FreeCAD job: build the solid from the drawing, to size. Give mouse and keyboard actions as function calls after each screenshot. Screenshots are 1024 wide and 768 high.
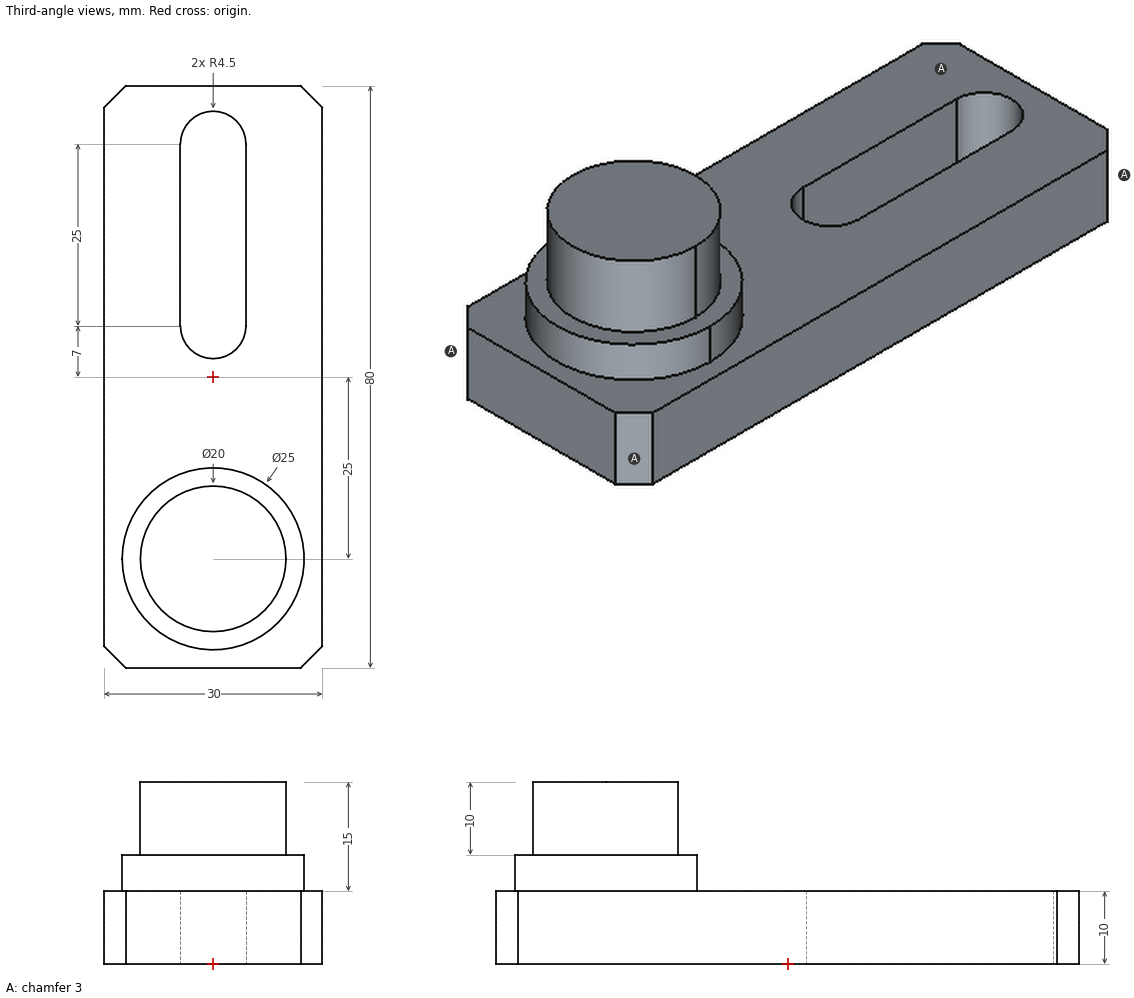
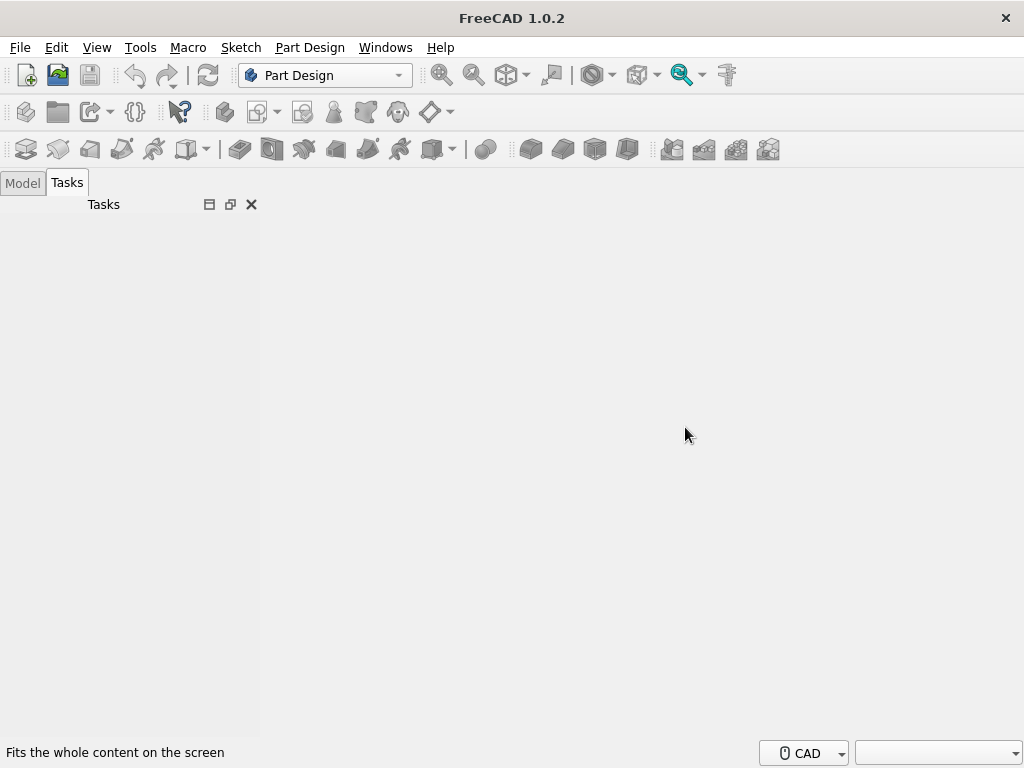
click(26, 76)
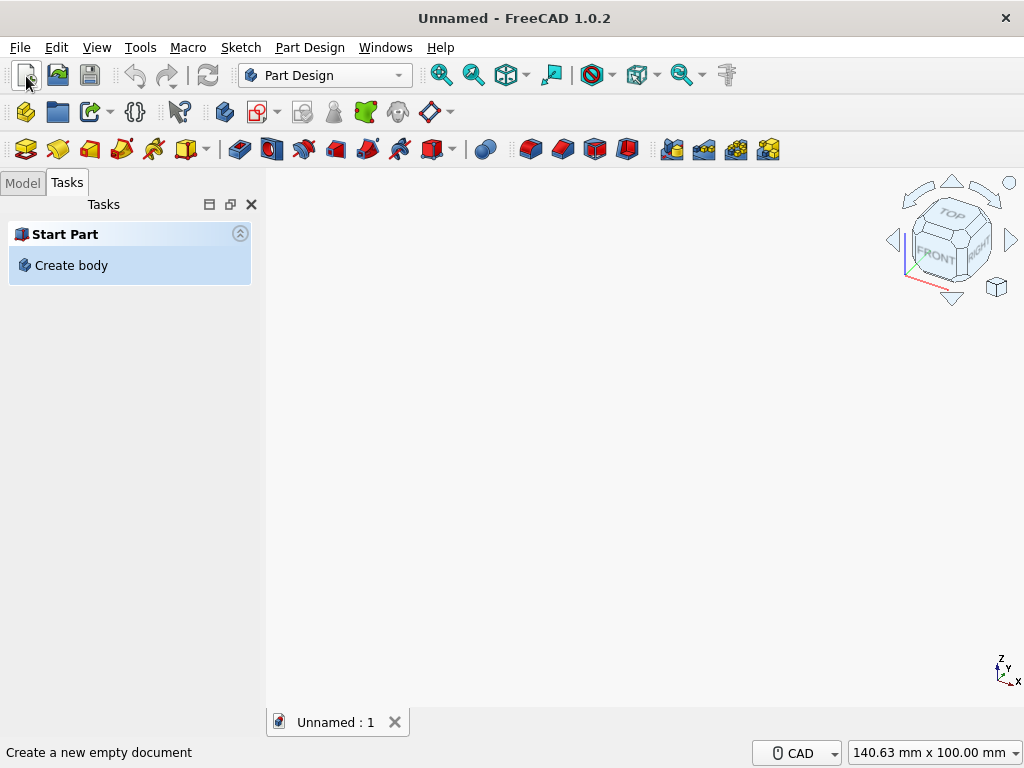
click(258, 112)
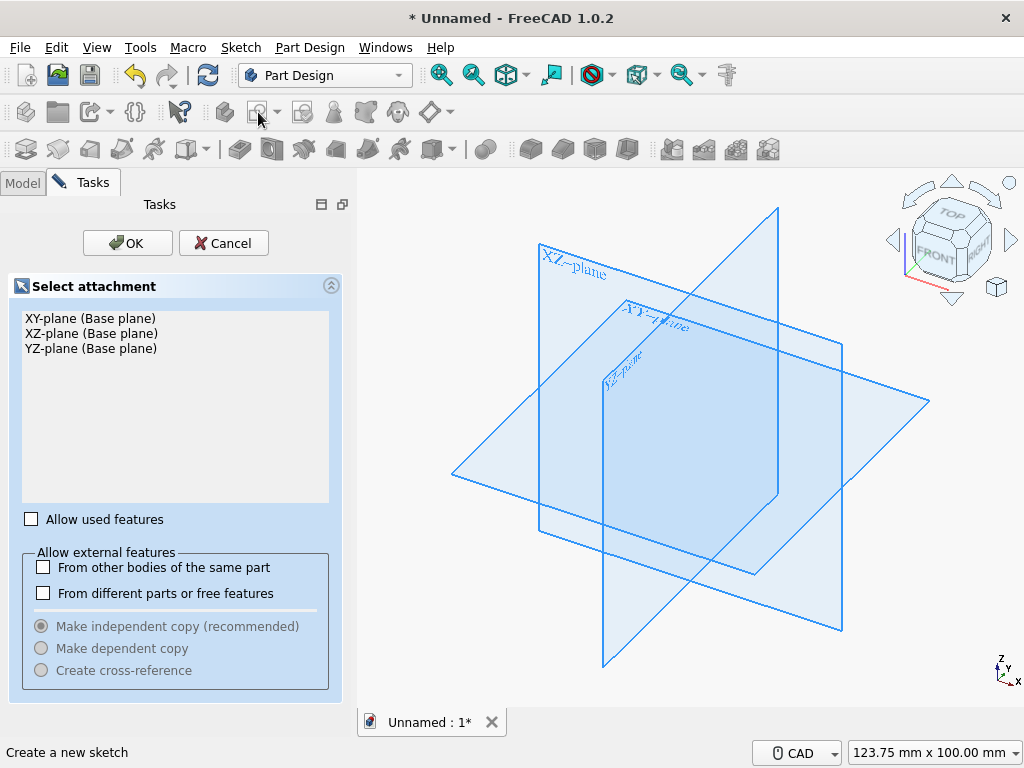
click(82, 318)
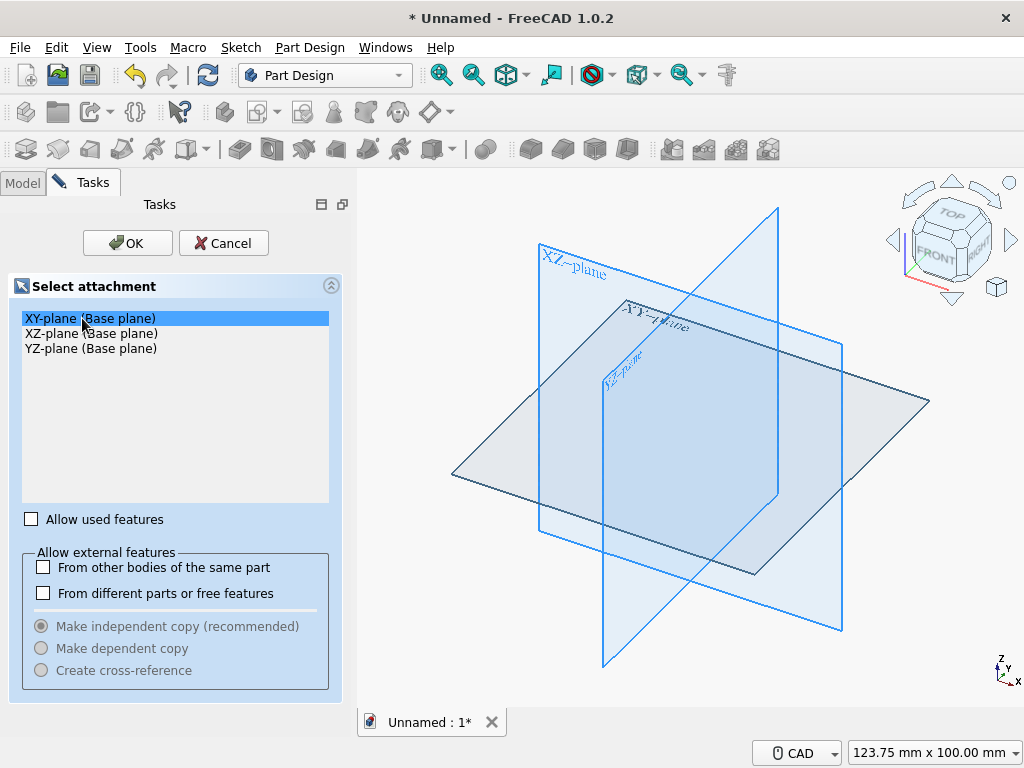
click(128, 243)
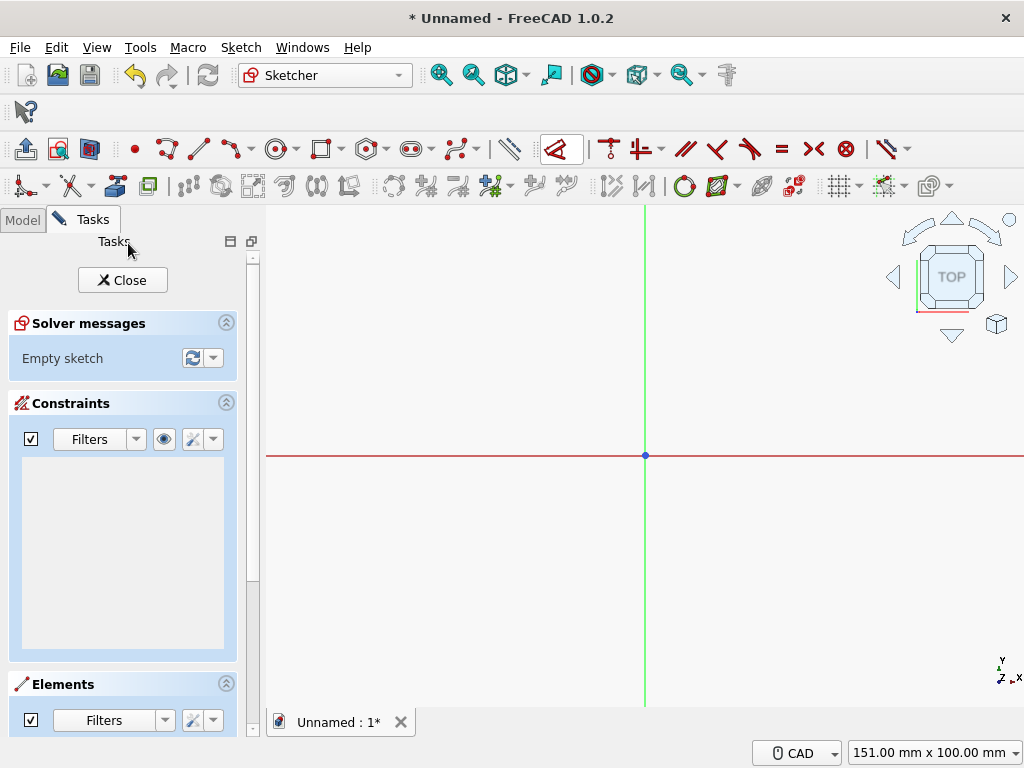
scroll(294, 456, down, 1)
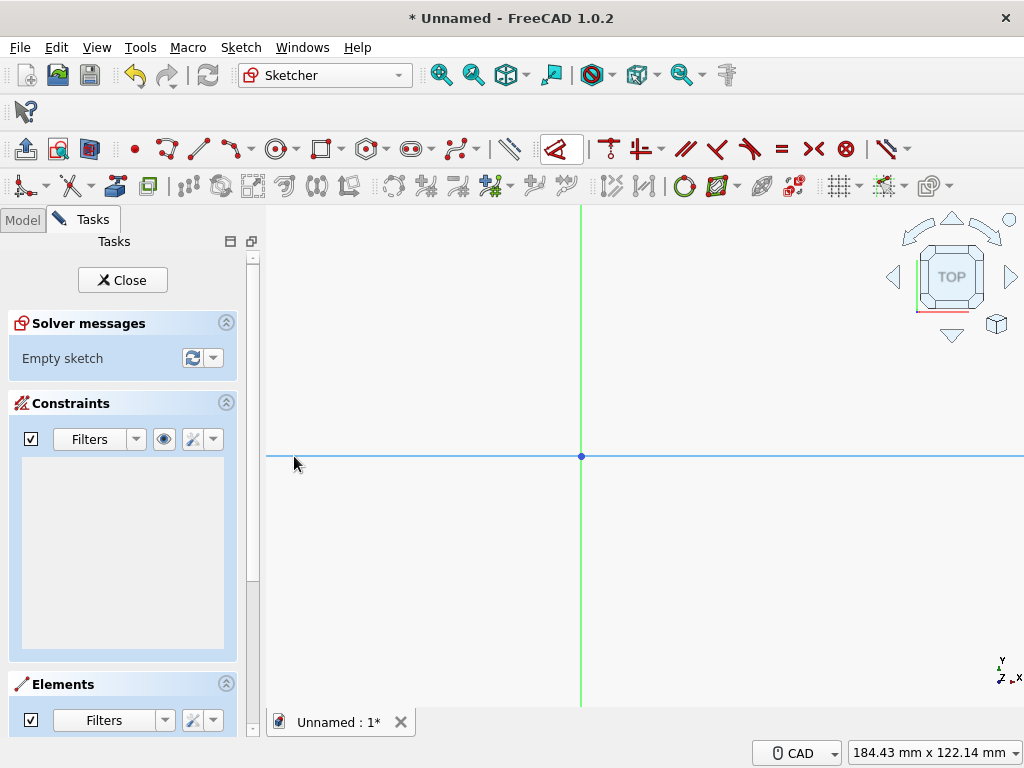
click(344, 150)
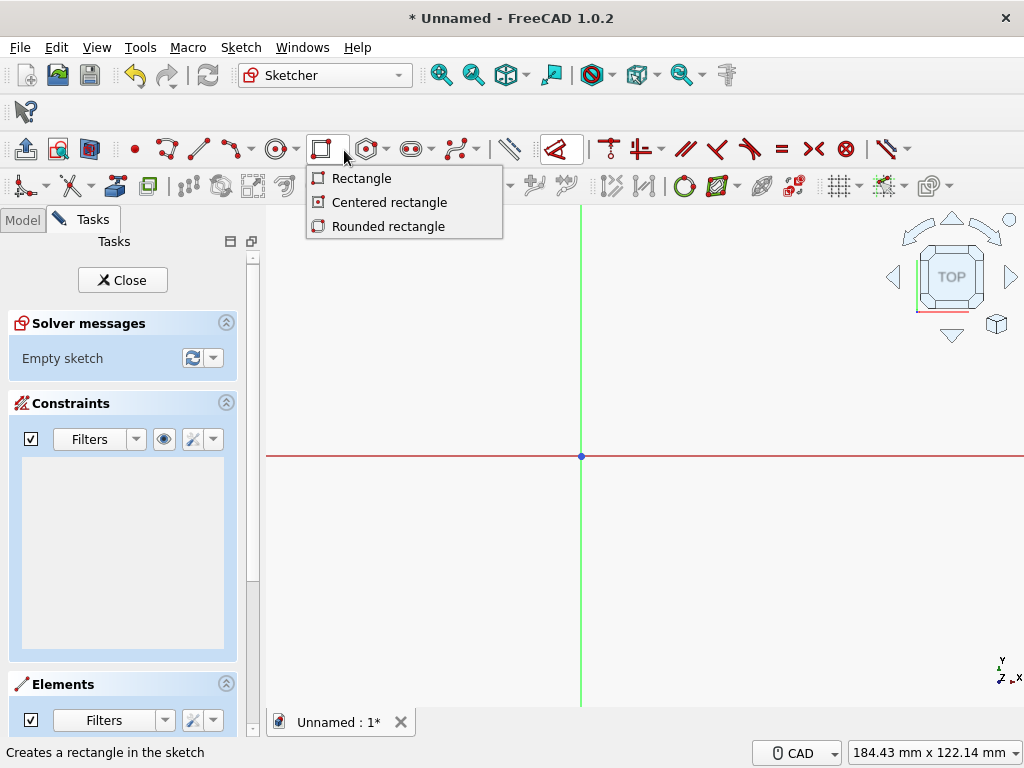
click(404, 202)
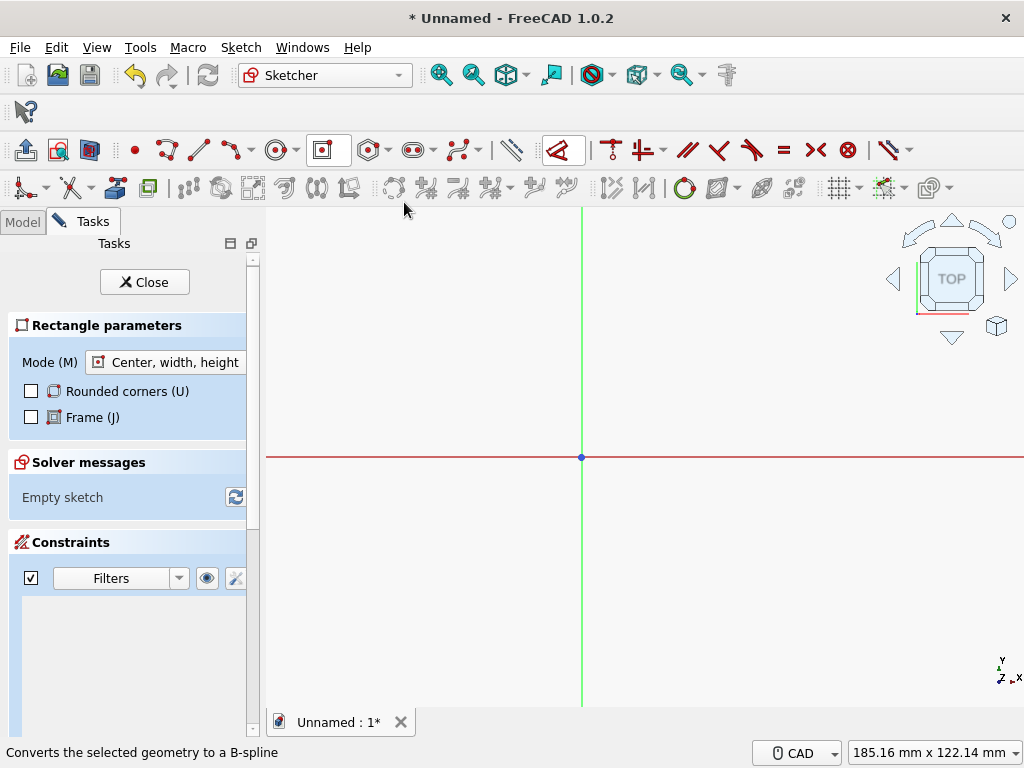
click(582, 457)
move(643, 293)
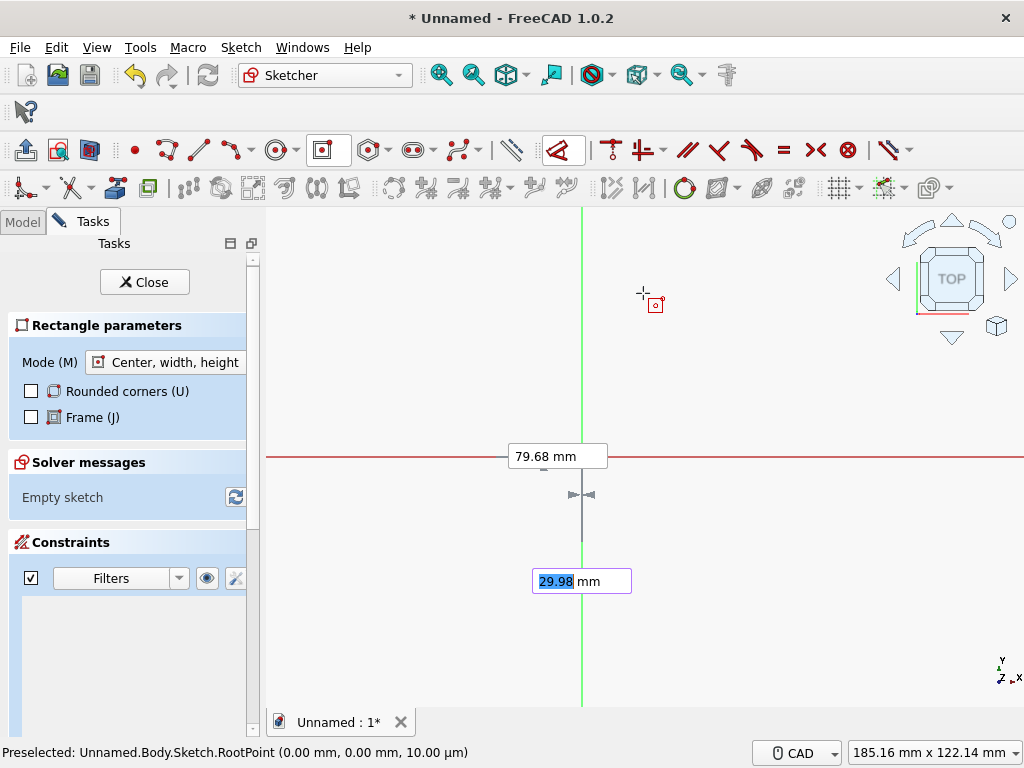
text(30)
key(Tab)
text(80)
key(Return)
key(Escape)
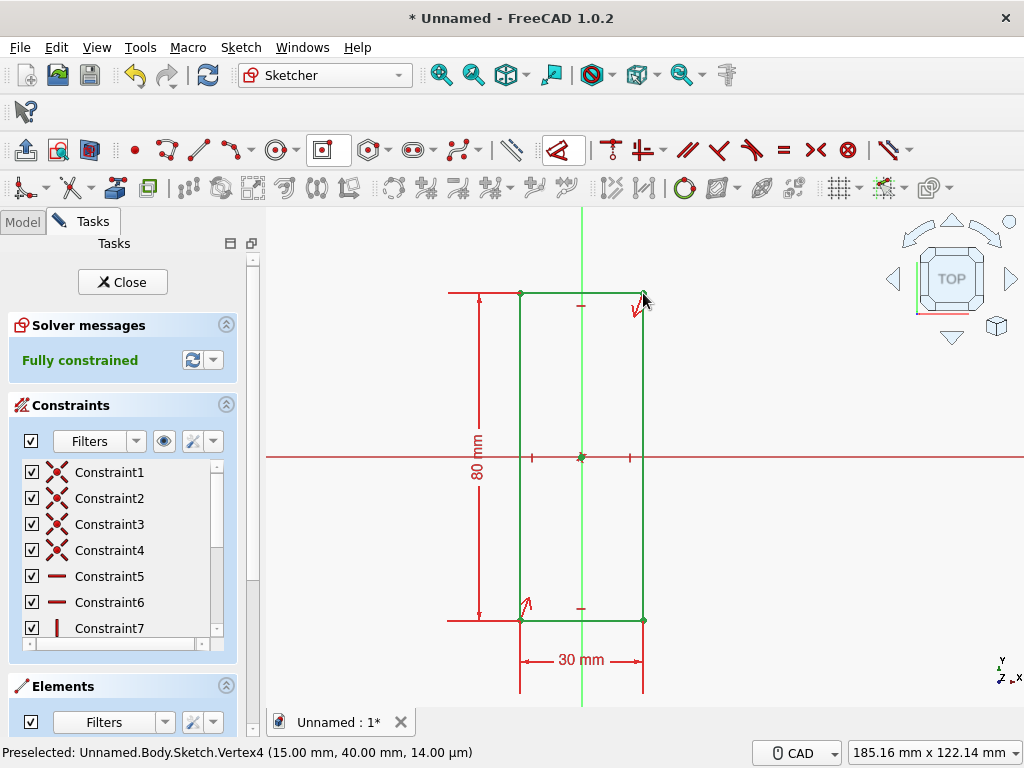
click(123, 282)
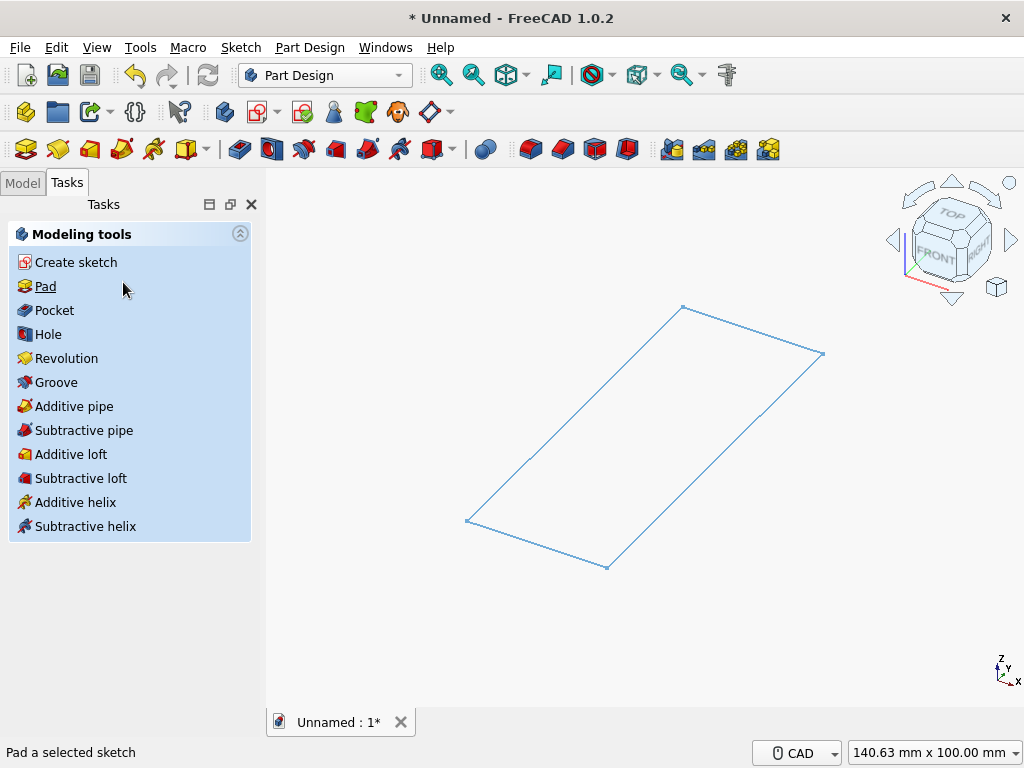
click(26, 150)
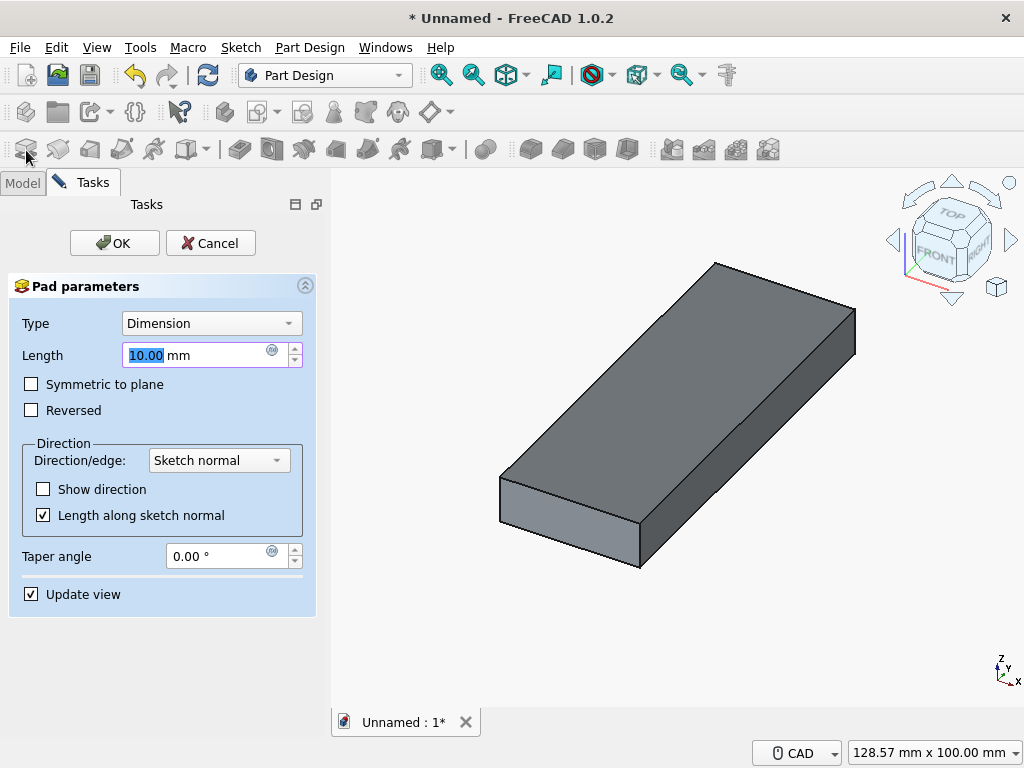
text(10)
key(Tab)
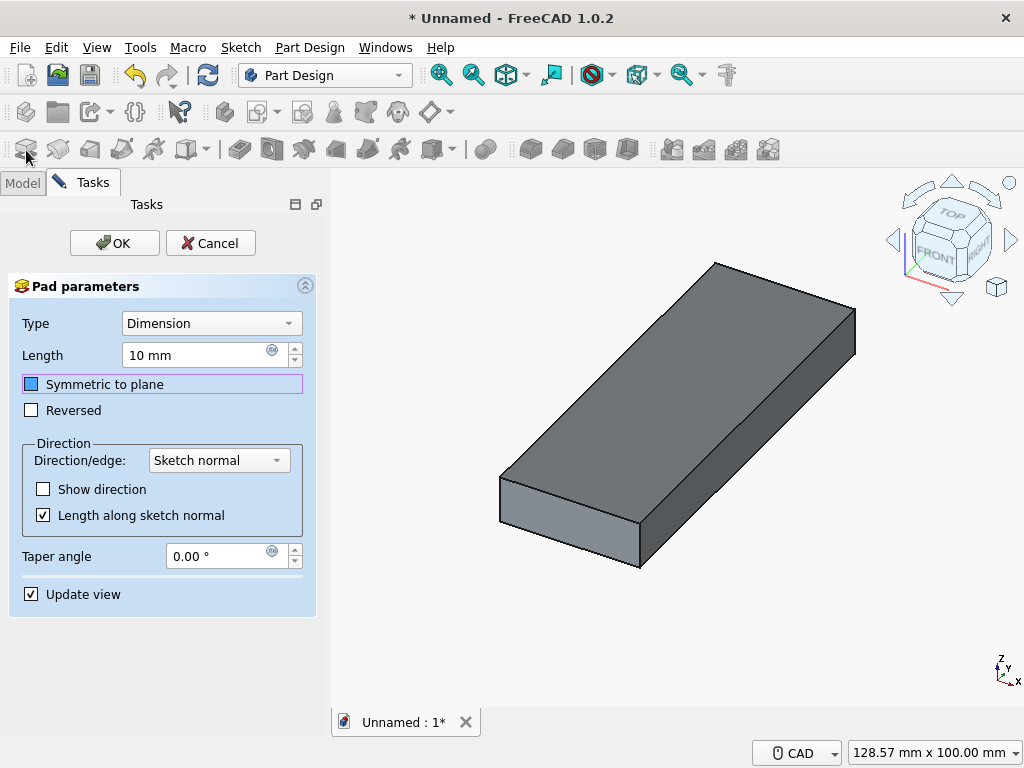
click(115, 243)